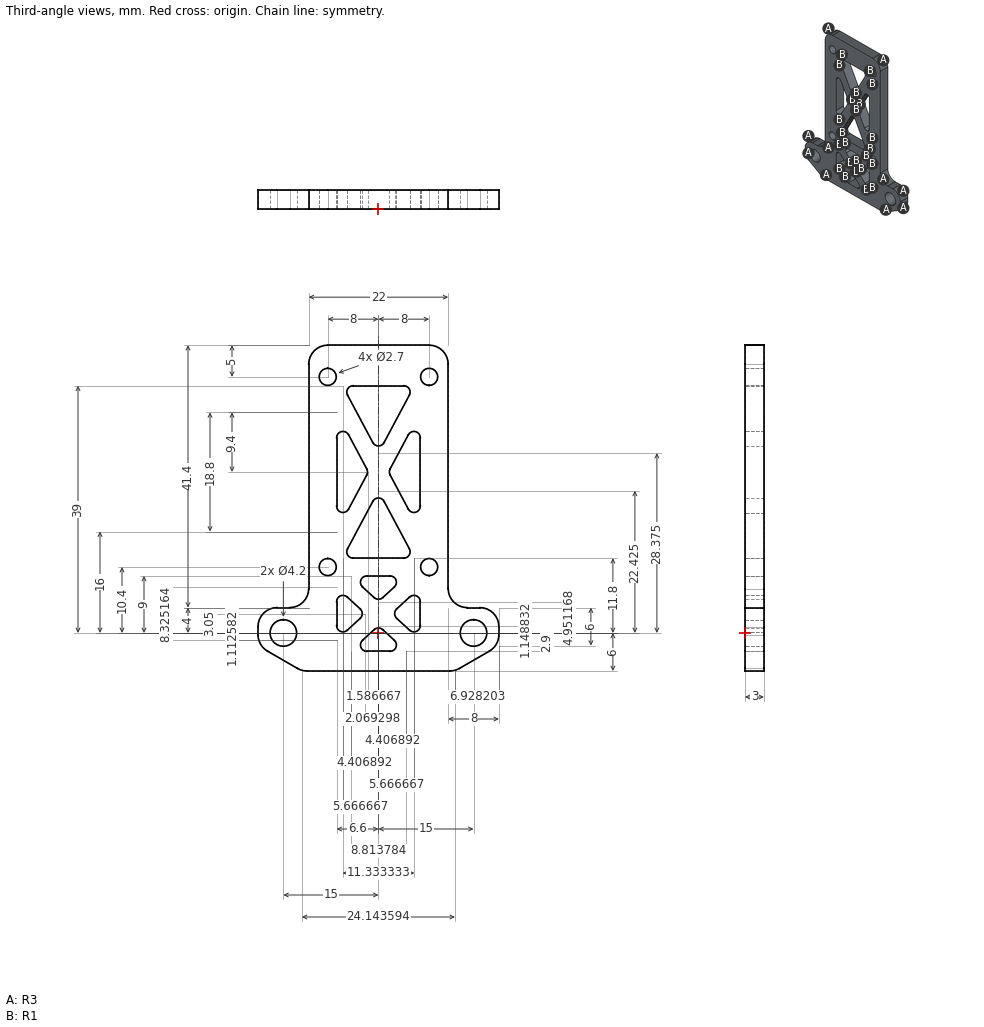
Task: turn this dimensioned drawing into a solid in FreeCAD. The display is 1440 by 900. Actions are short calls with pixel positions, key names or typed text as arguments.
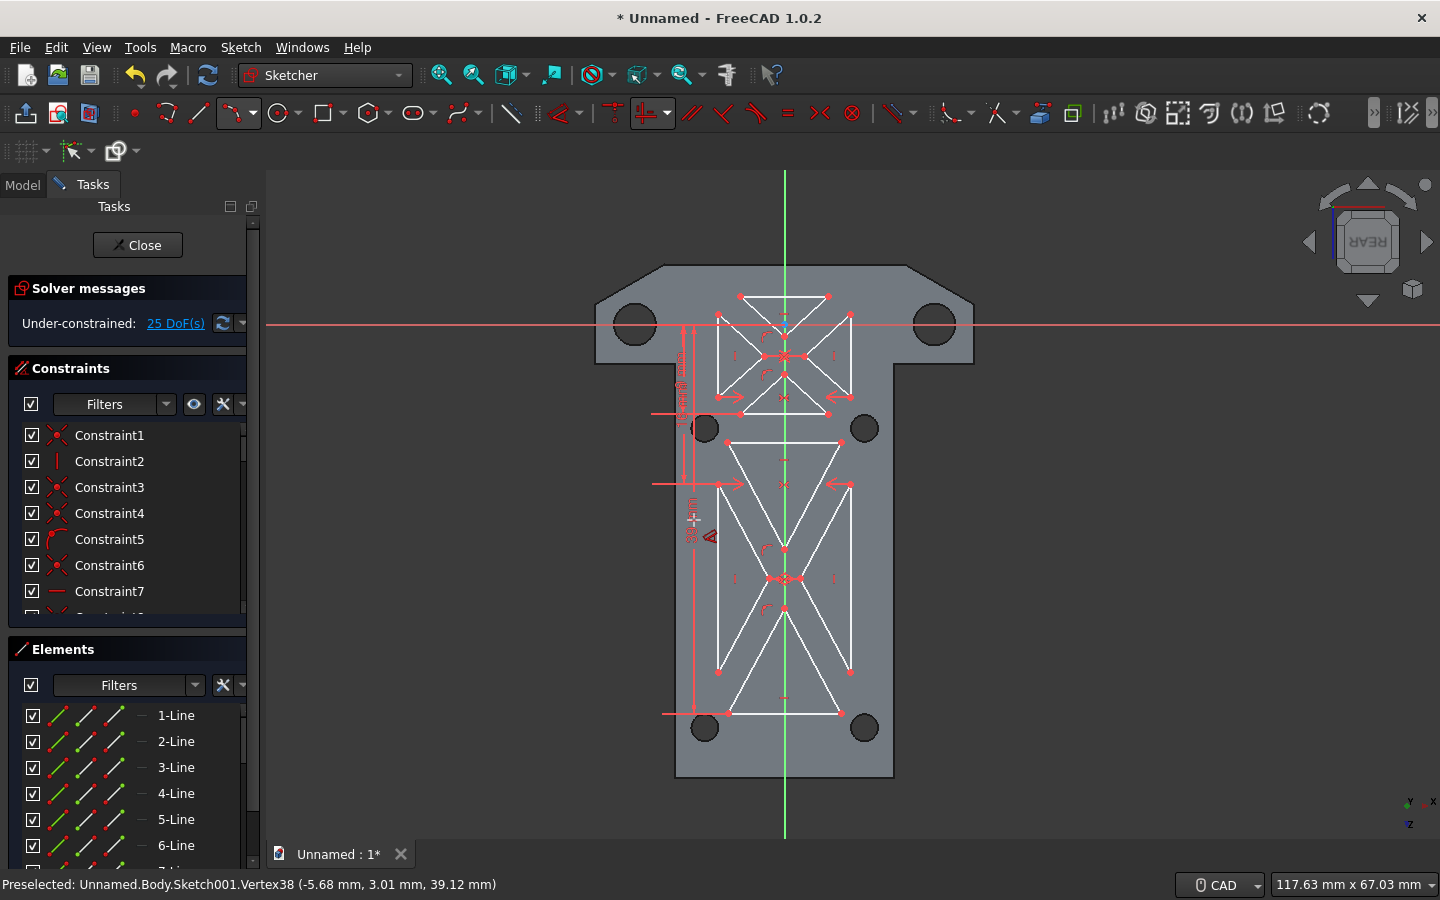
click(718, 541)
click(684, 579)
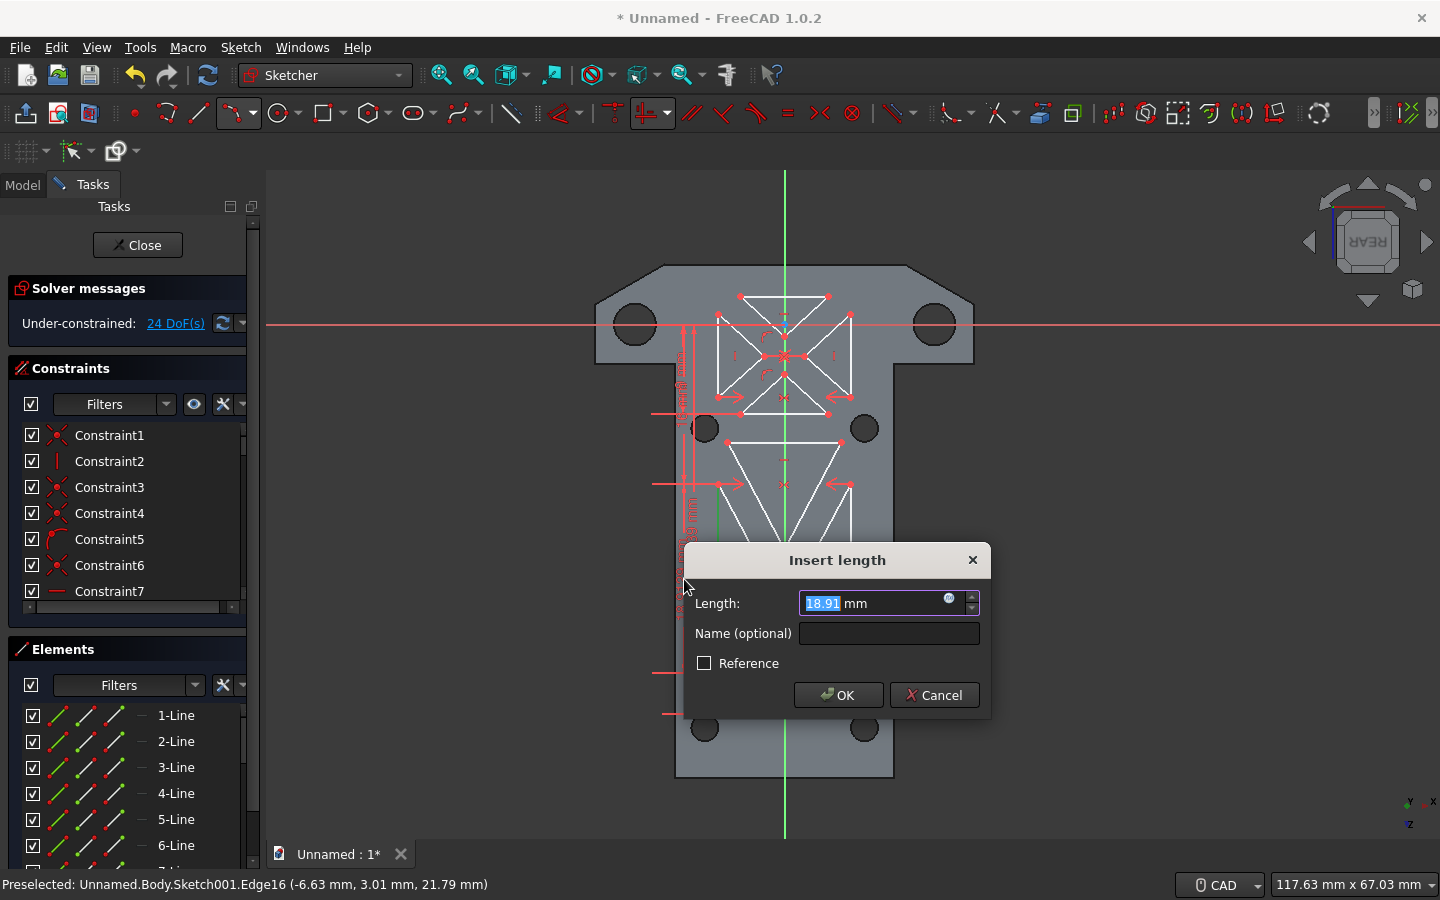
text(18.8)
key(Return)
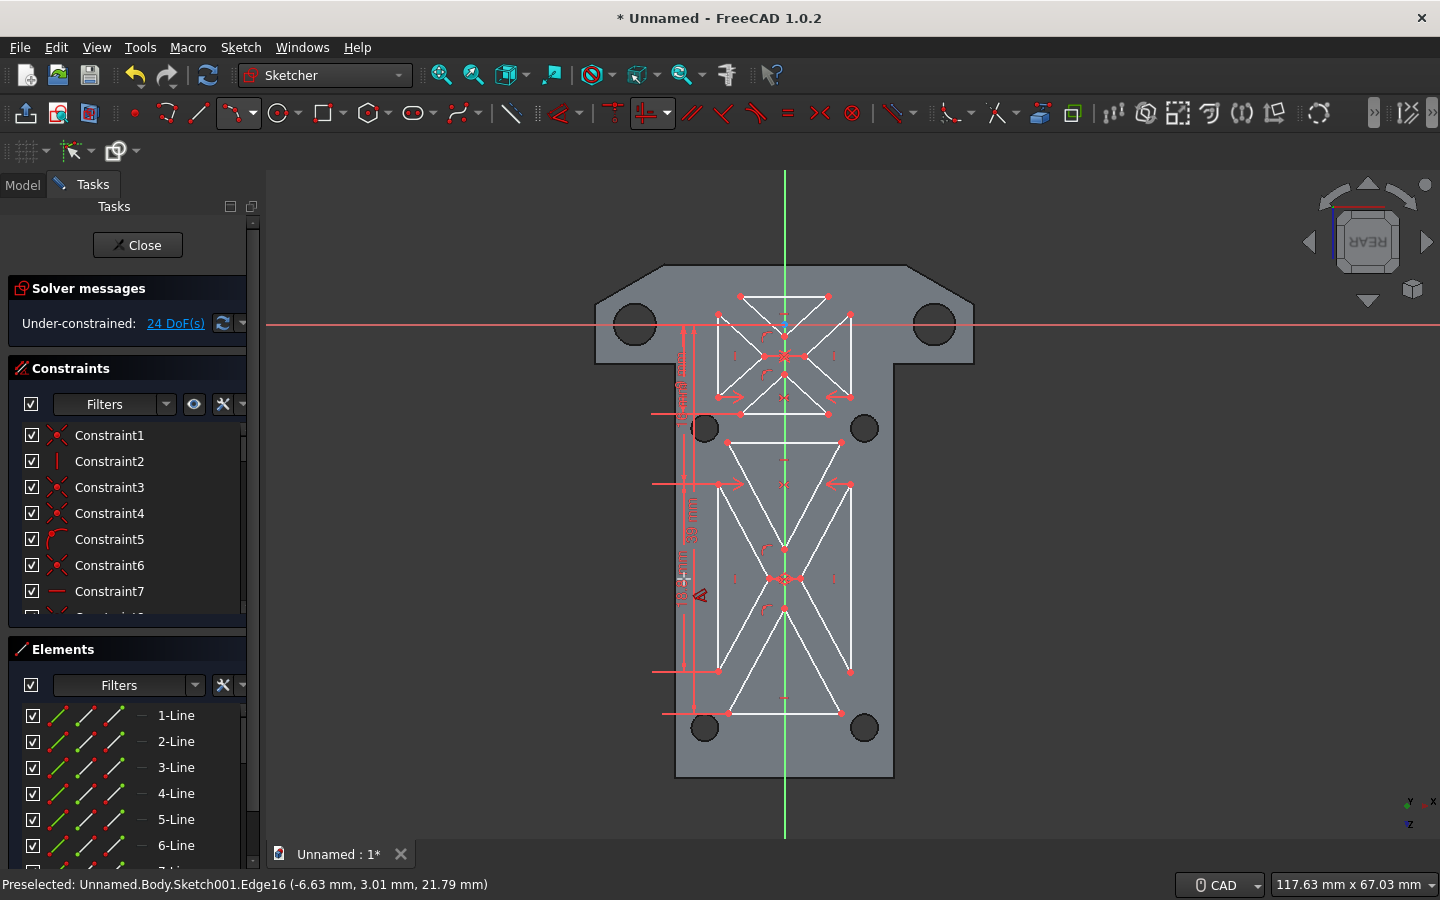
click(851, 616)
click(885, 579)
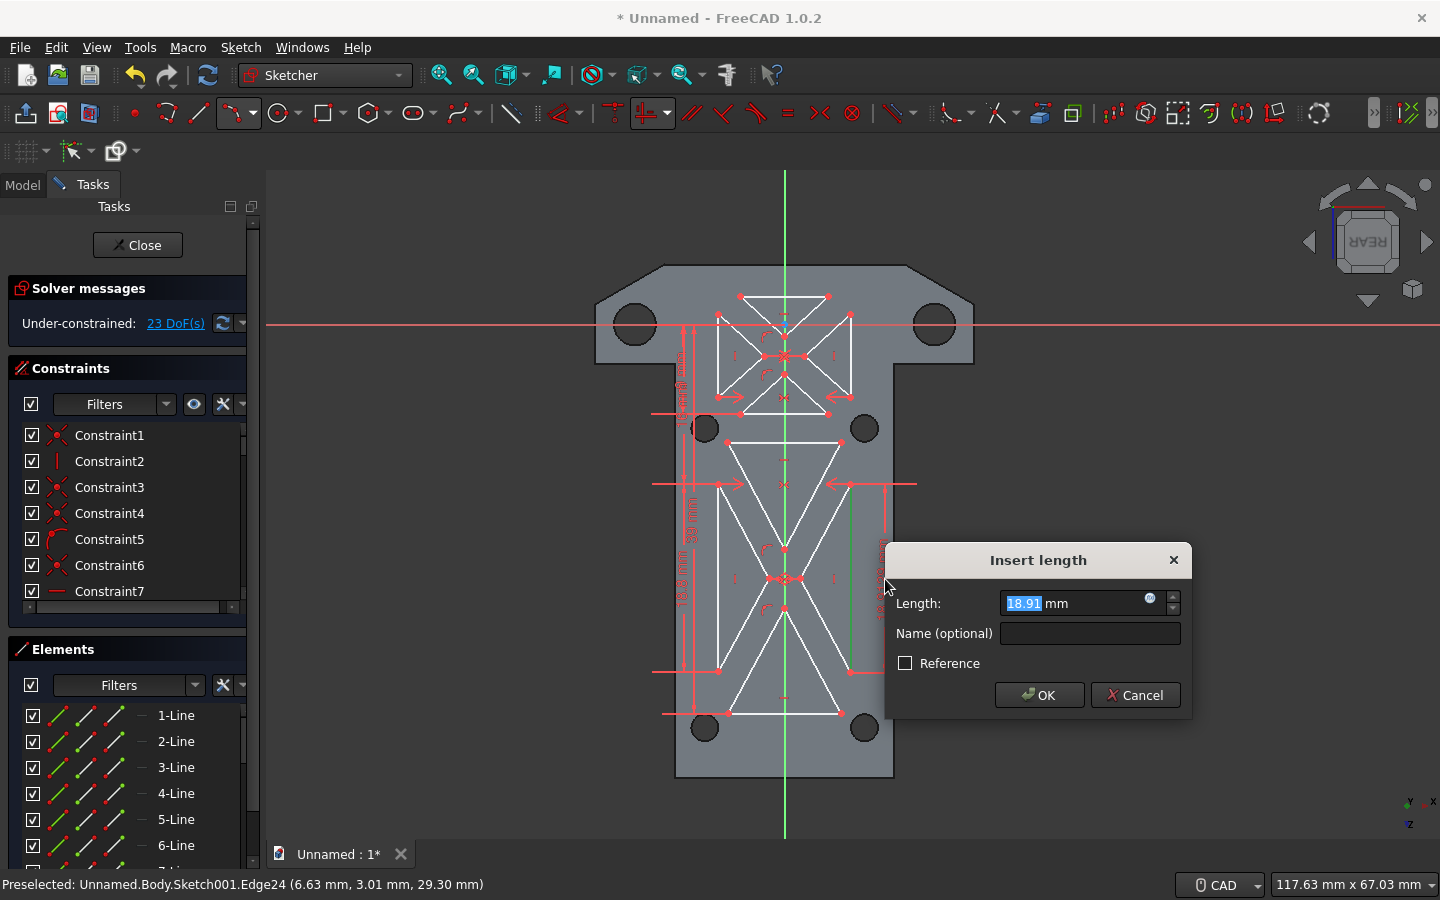
text(18.8)
key(Return)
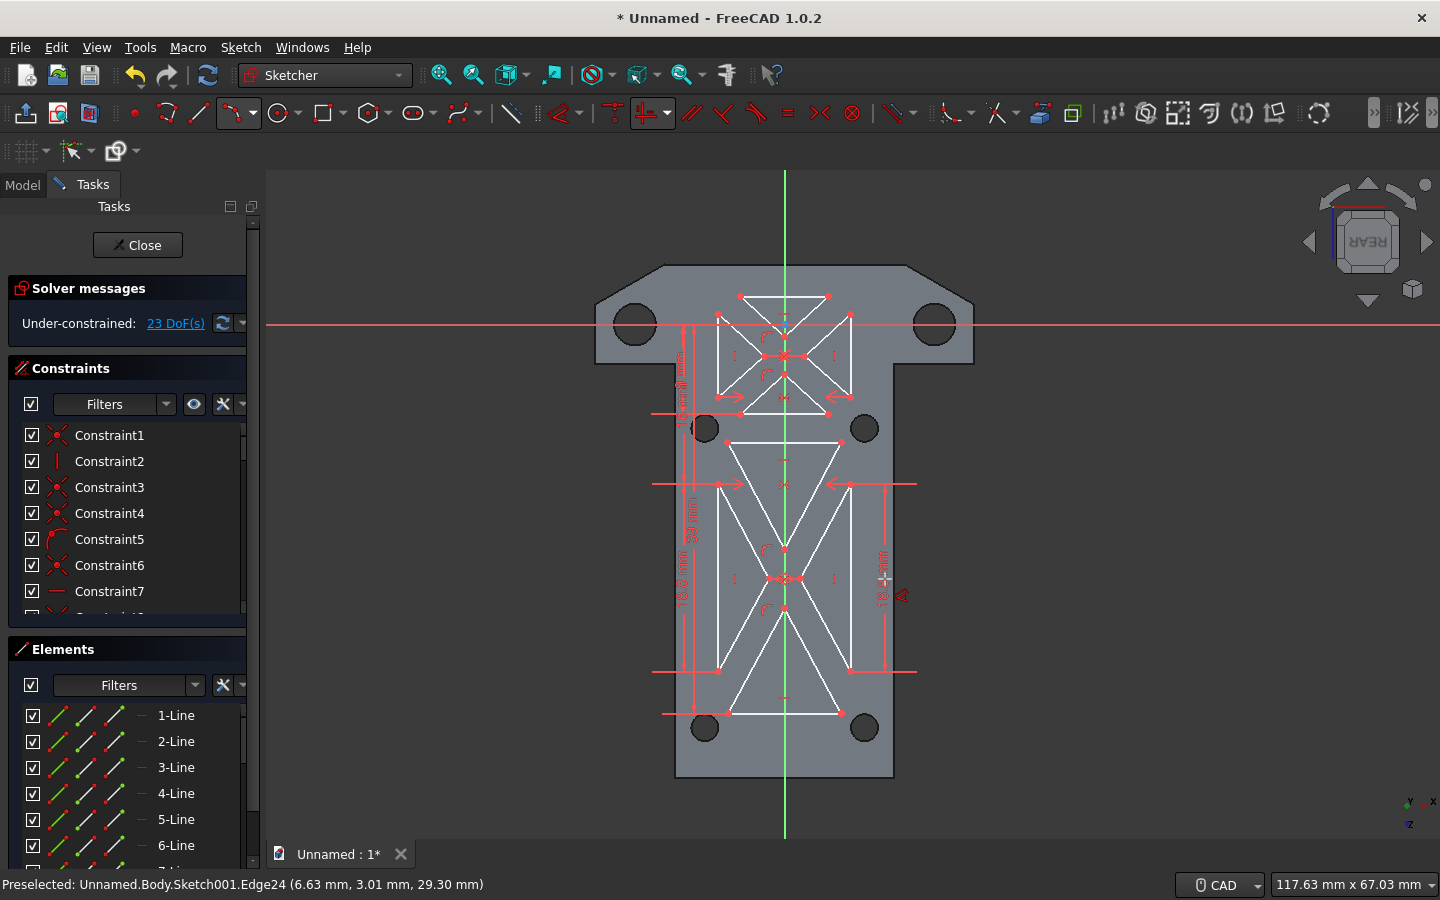
click(718, 314)
click(752, 280)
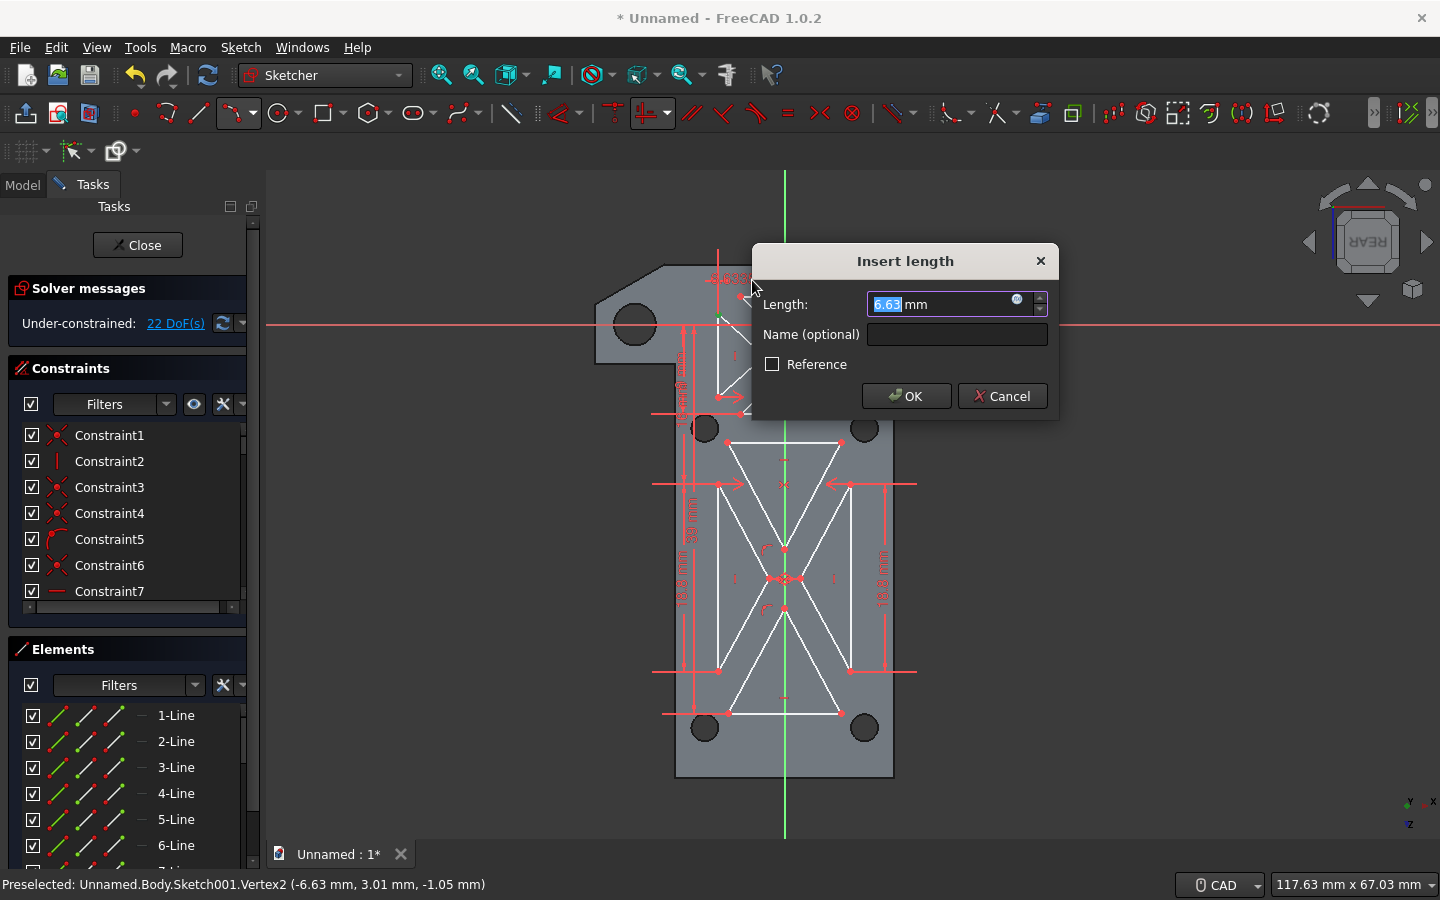
text(6.6)
key(Return)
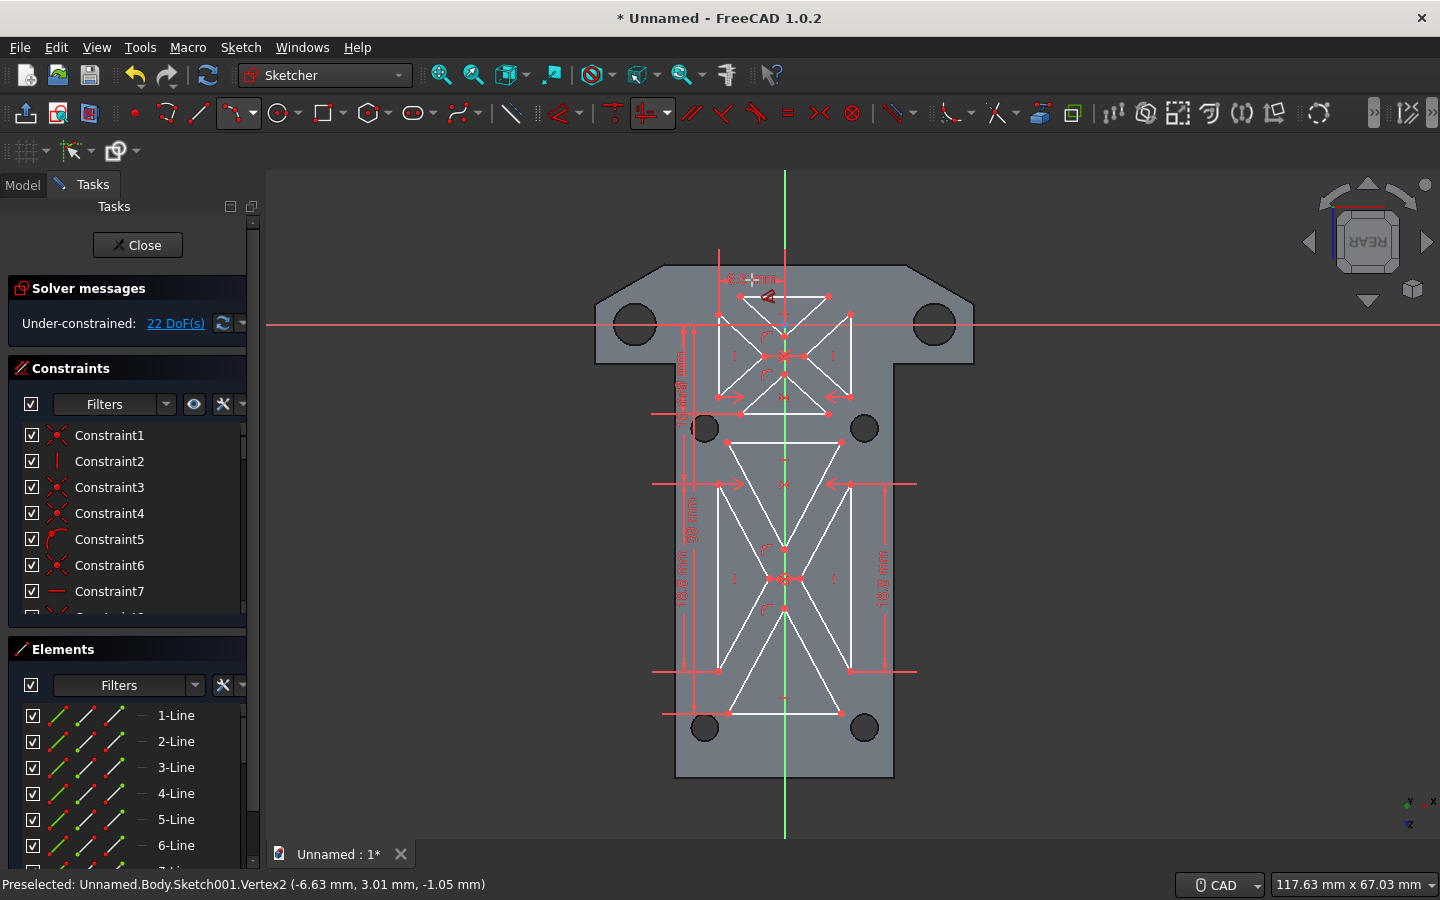
scroll(828, 297, up, 2)